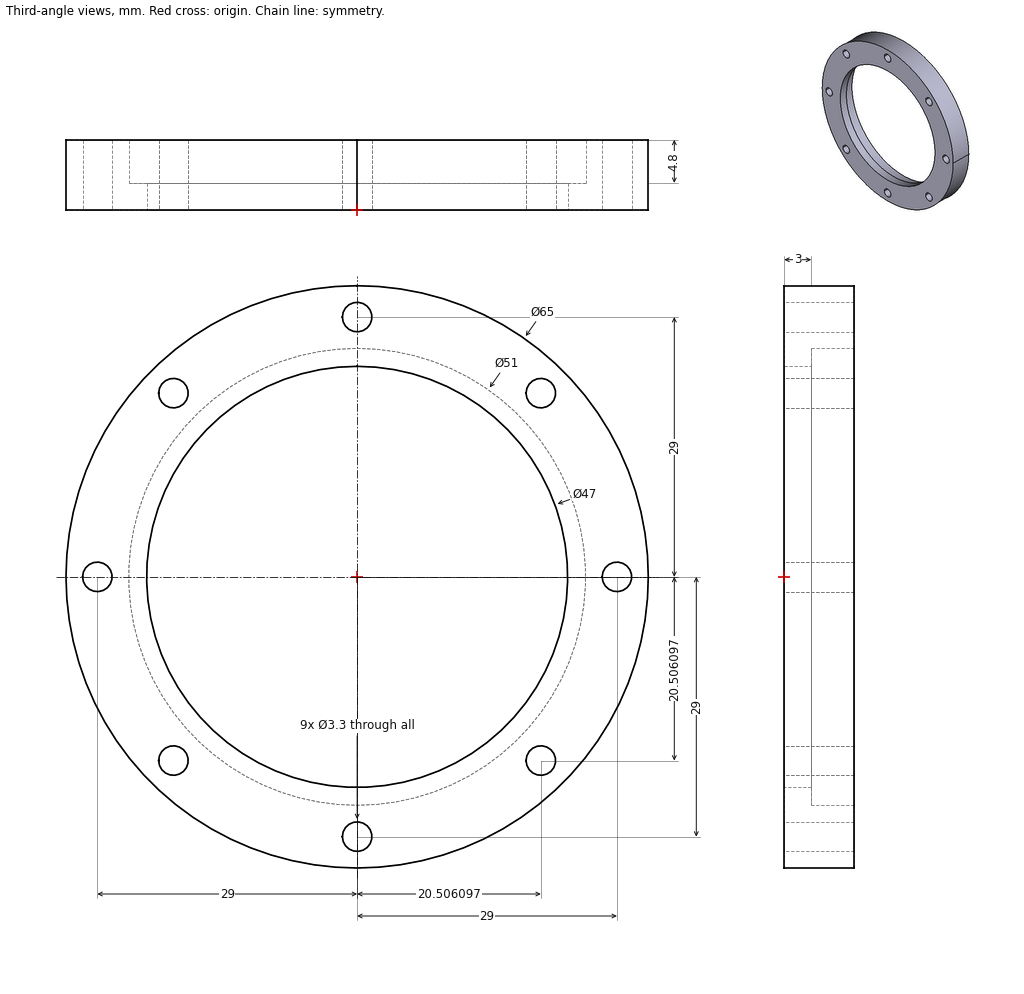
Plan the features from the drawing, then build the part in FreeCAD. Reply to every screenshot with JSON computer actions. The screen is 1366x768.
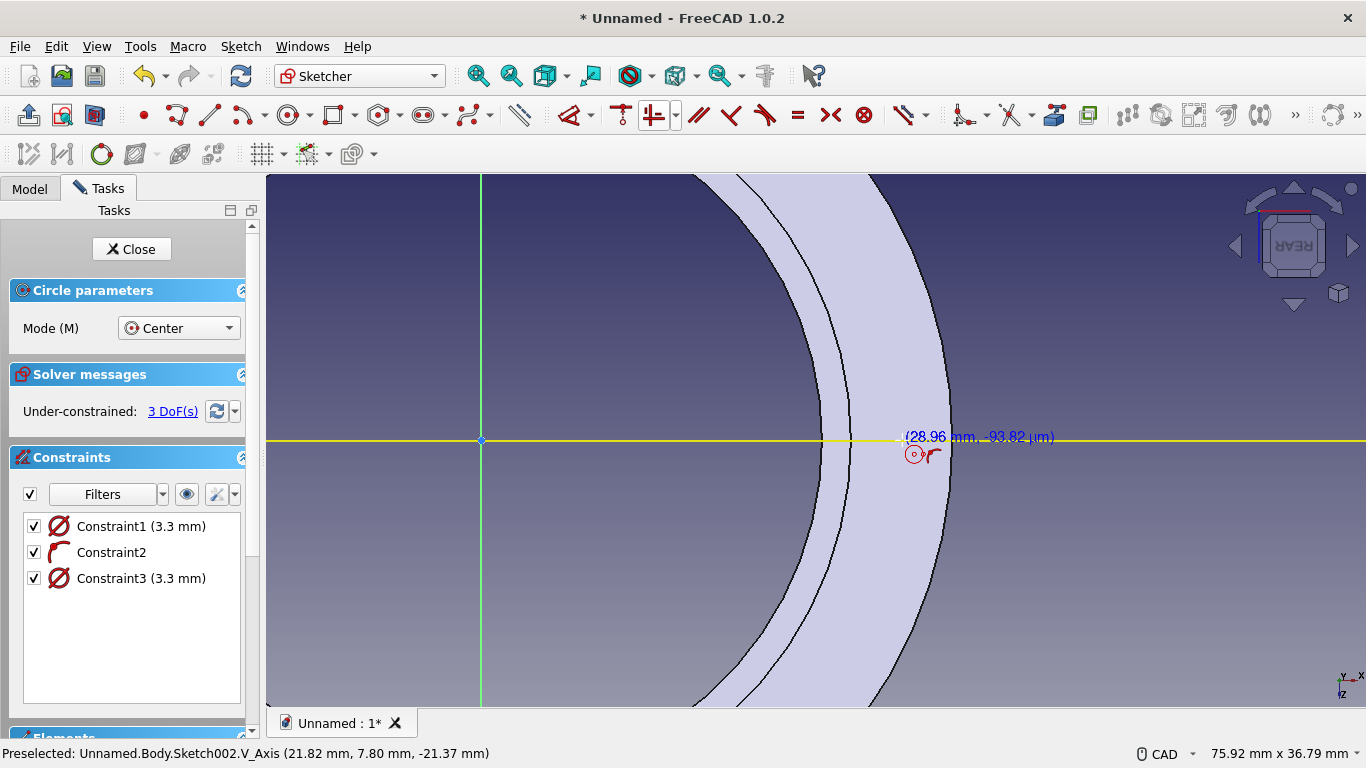
{"action": "left_click", "coordinate": [902, 440]}
{"action": "mouse_move", "coordinate": [919, 424]}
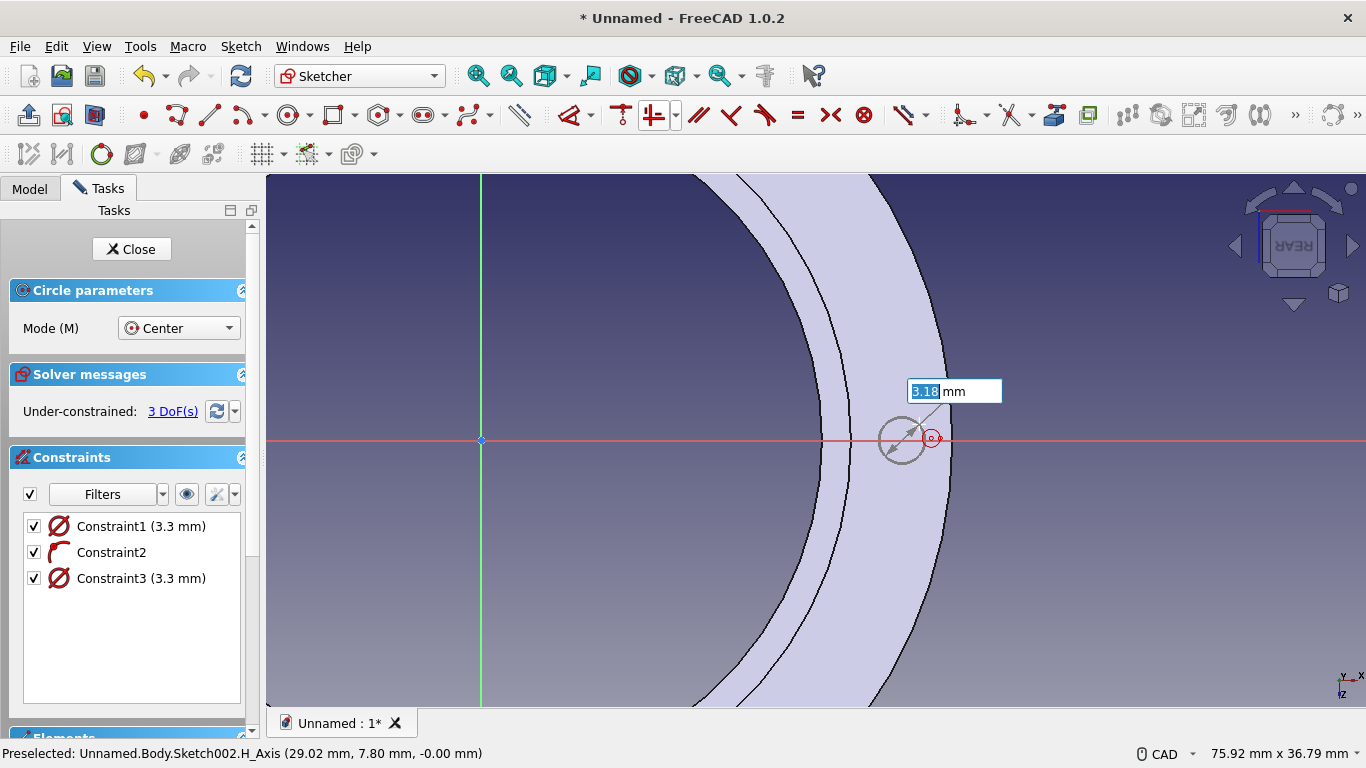
{"action": "type", "text": "3.3"}
{"action": "key", "text": "Return"}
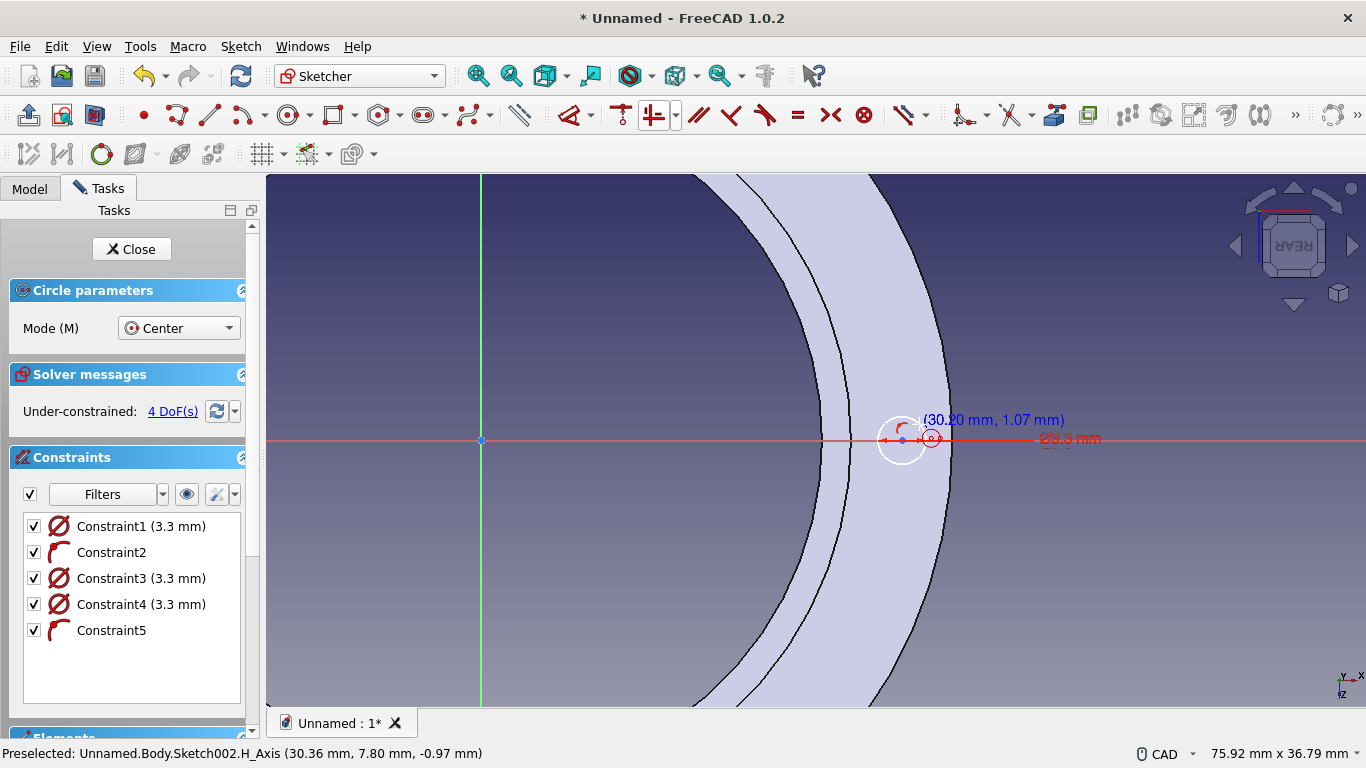
{"action": "scroll", "coordinate": [902, 441], "scroll_direction": "down", "scroll_amount": 5}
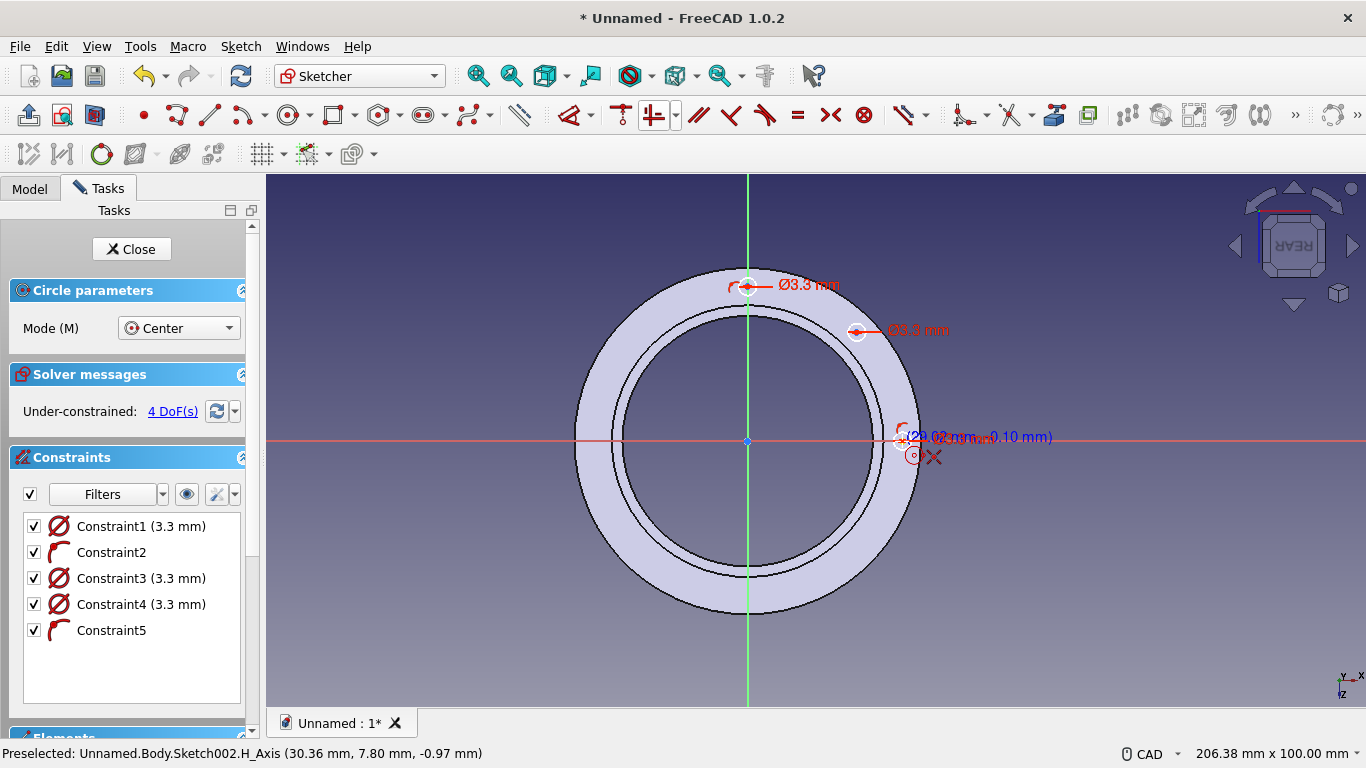
{"action": "scroll", "coordinate": [857, 550], "scroll_direction": "up", "scroll_amount": 5}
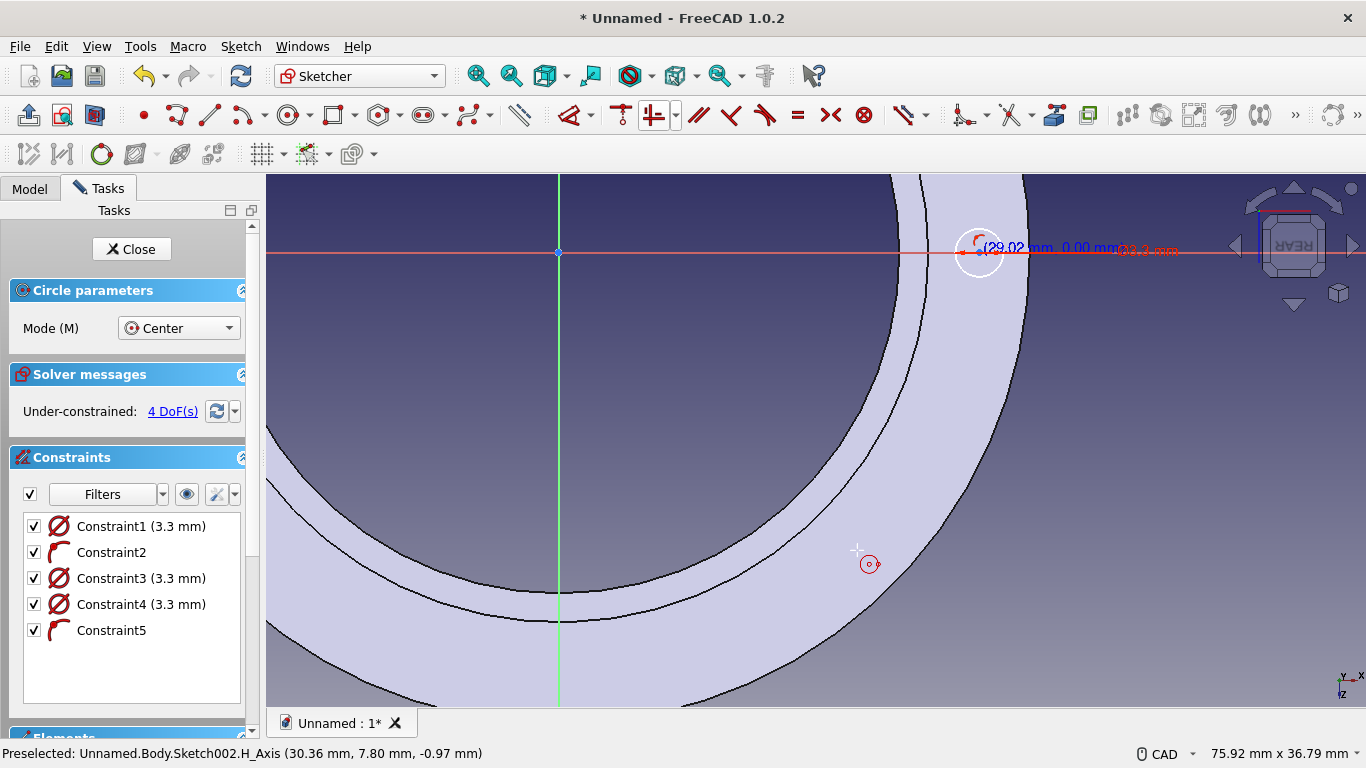
{"action": "left_click", "coordinate": [856, 550]}
{"action": "mouse_move", "coordinate": [873, 533]}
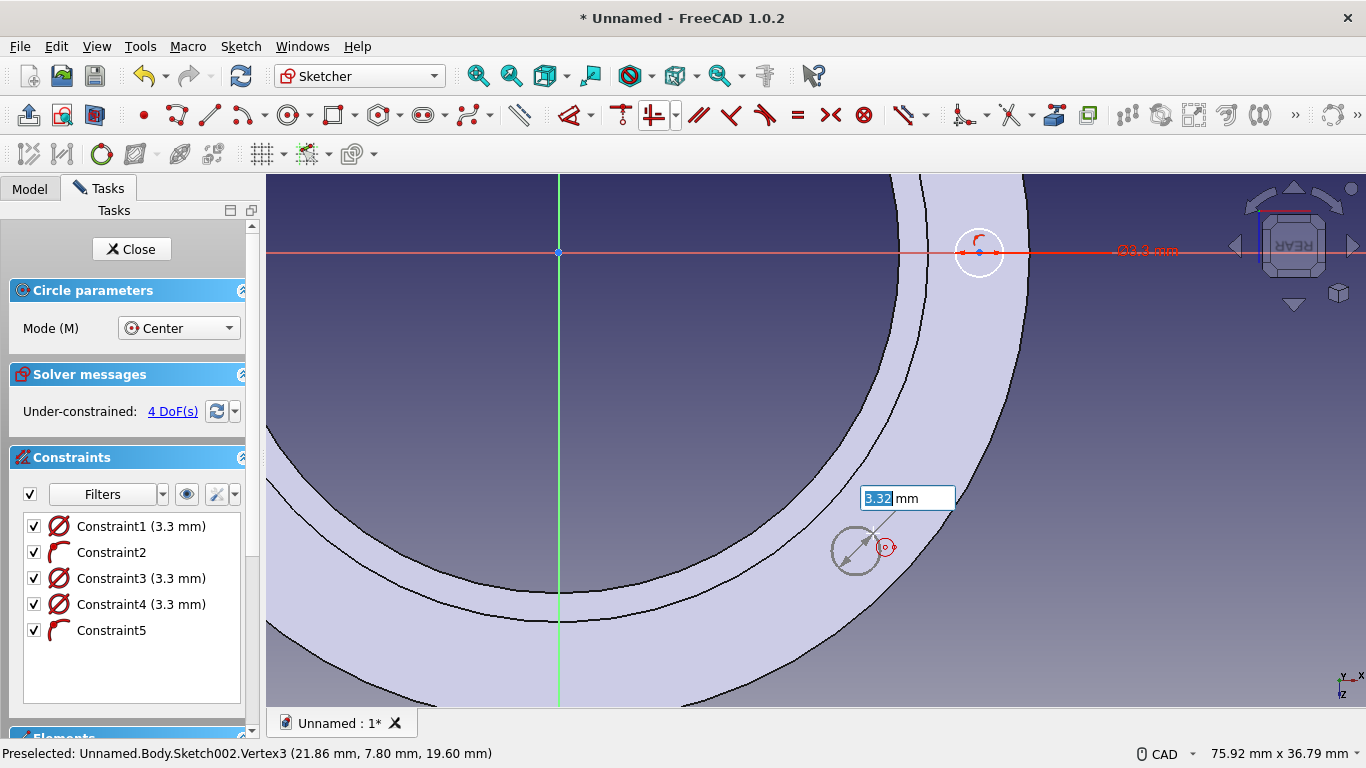
{"action": "type", "text": "3.3"}
{"action": "key", "text": "Return"}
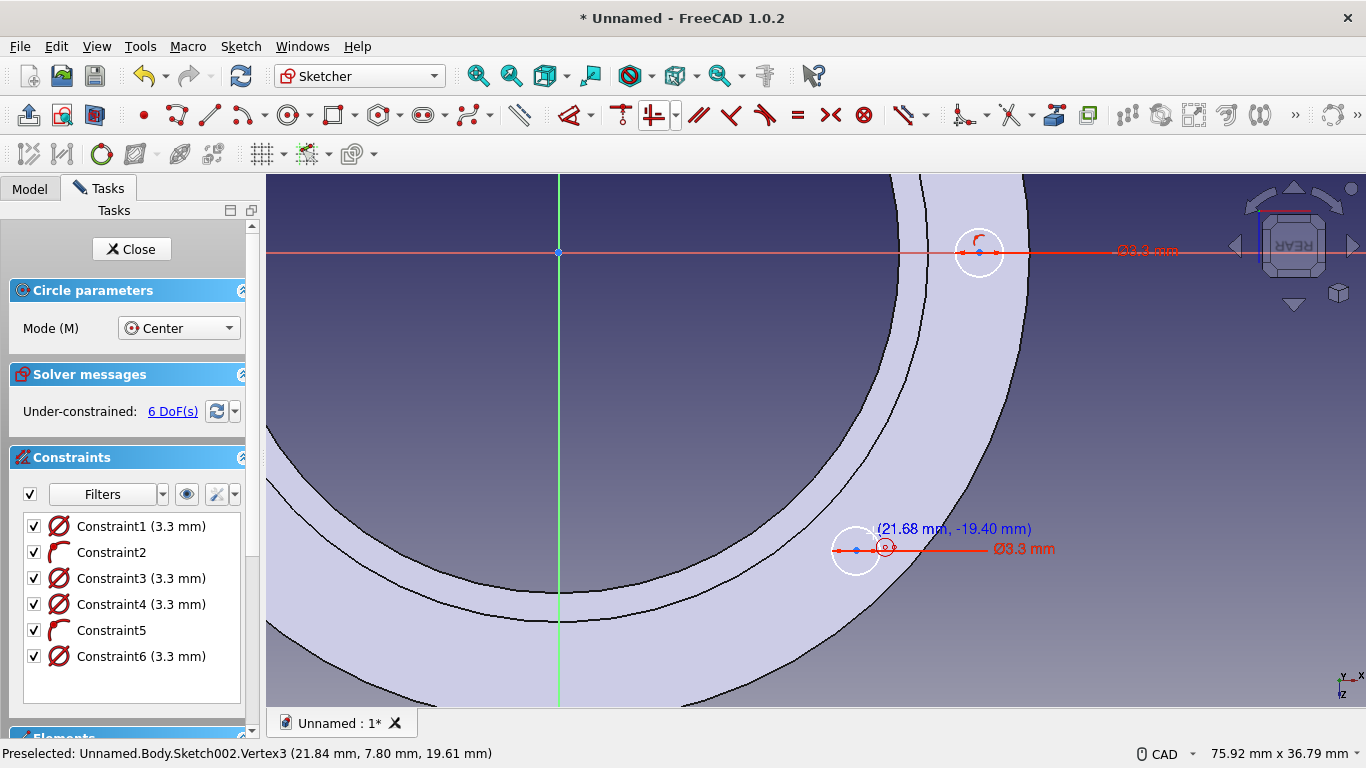
{"action": "left_click", "coordinate": [559, 673]}
{"action": "mouse_move", "coordinate": [576, 656]}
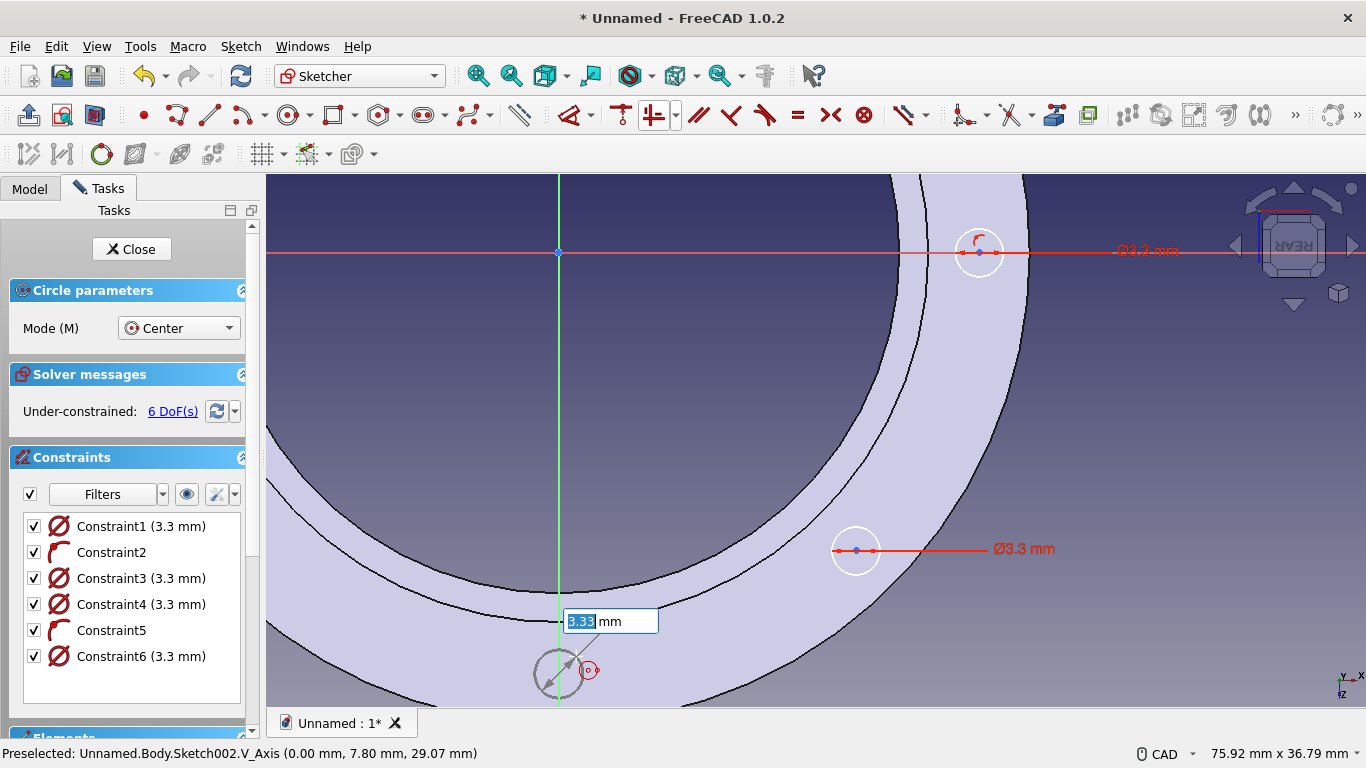
{"action": "type", "text": "3.3"}
{"action": "key", "text": "Return"}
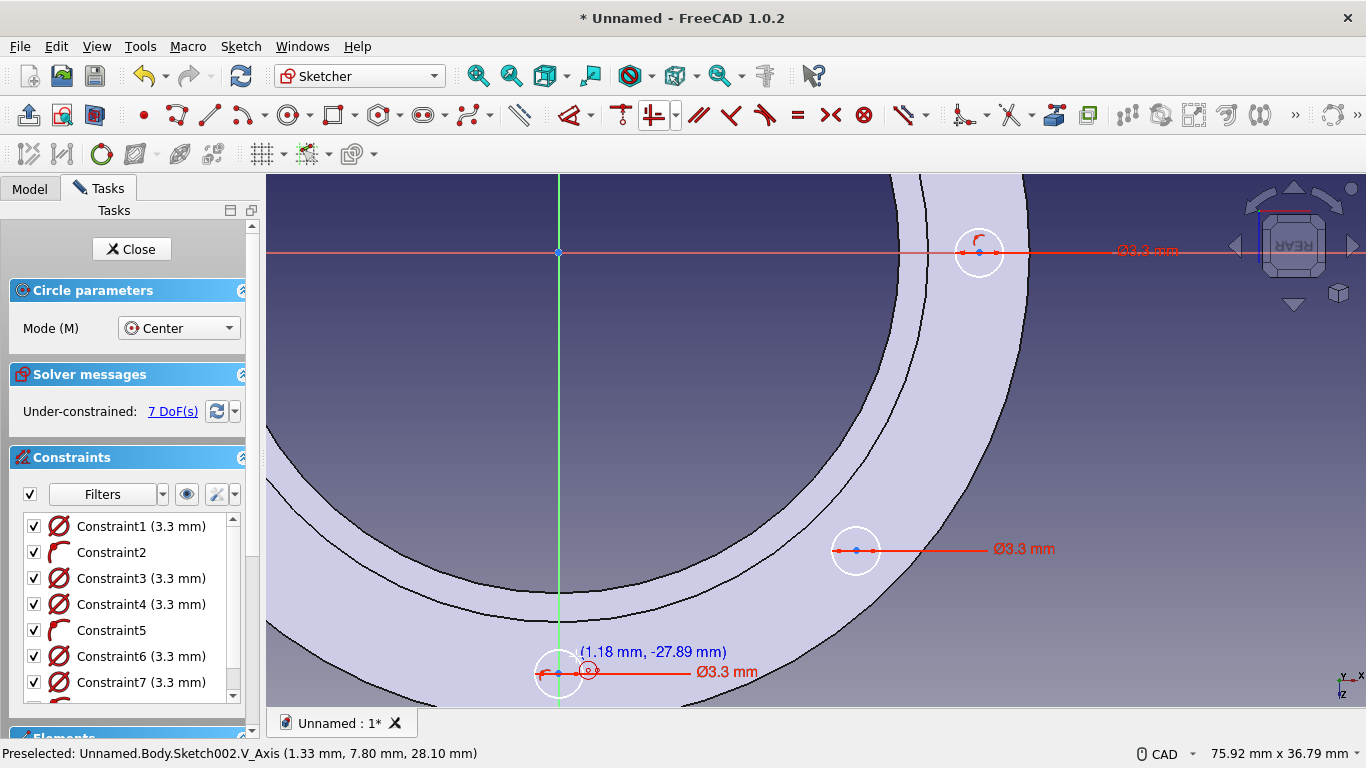
{"action": "scroll", "coordinate": [857, 550], "scroll_direction": "down", "scroll_amount": 5}